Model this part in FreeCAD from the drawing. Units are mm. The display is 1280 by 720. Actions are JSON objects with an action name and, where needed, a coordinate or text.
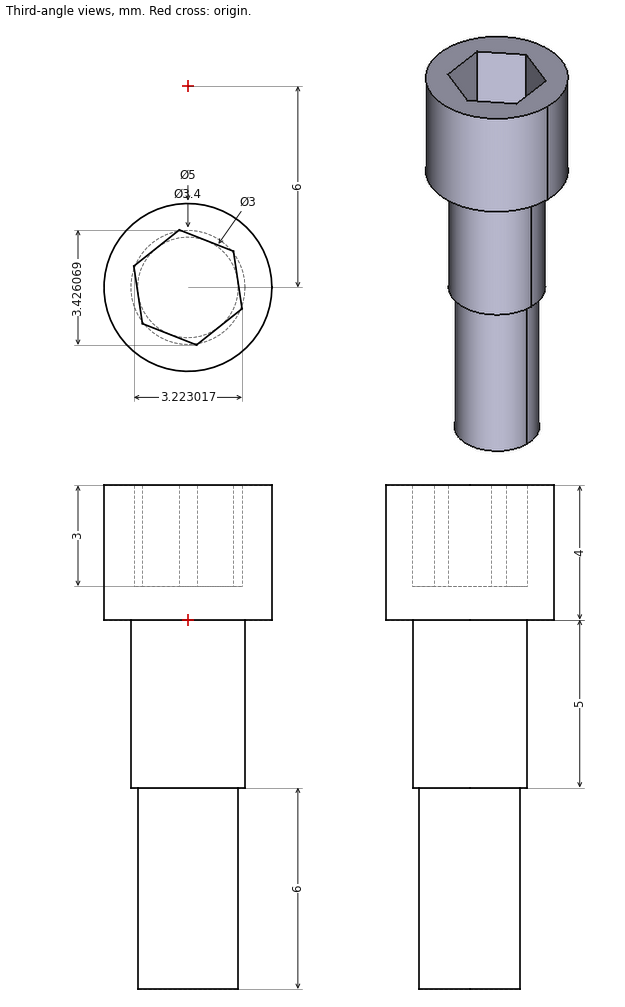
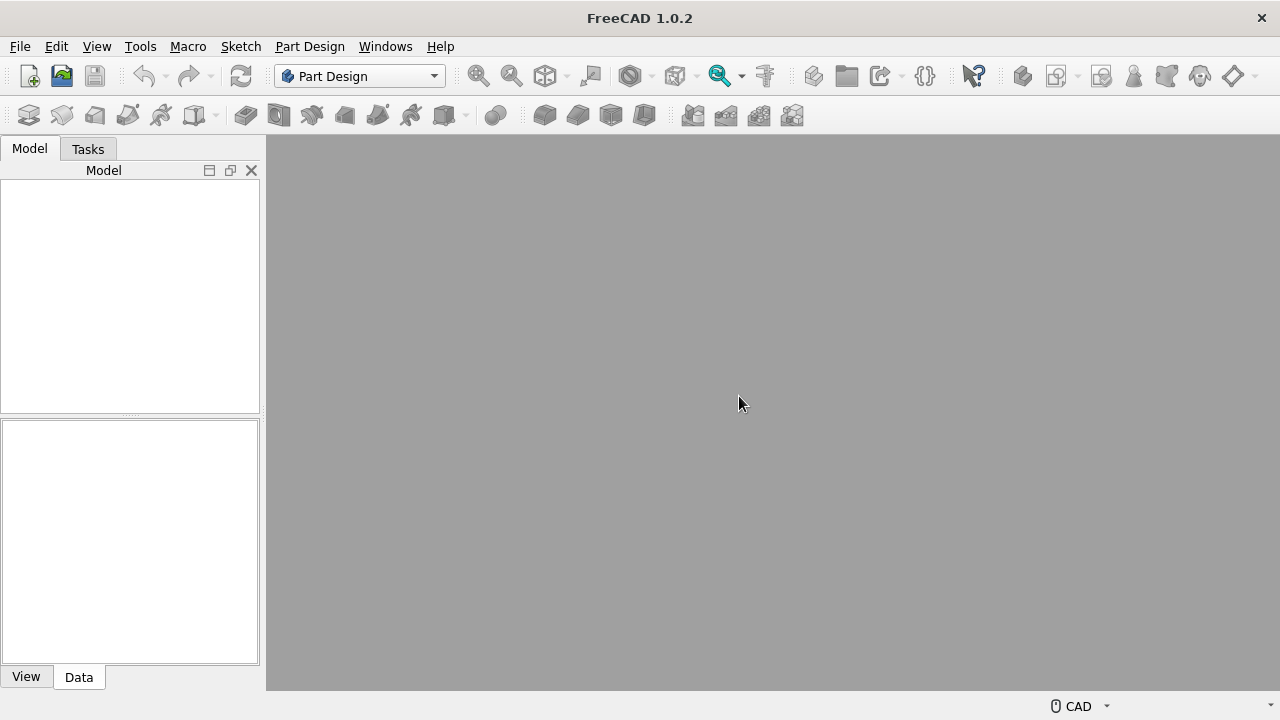
{"action": "left_click", "coordinate": [29, 76]}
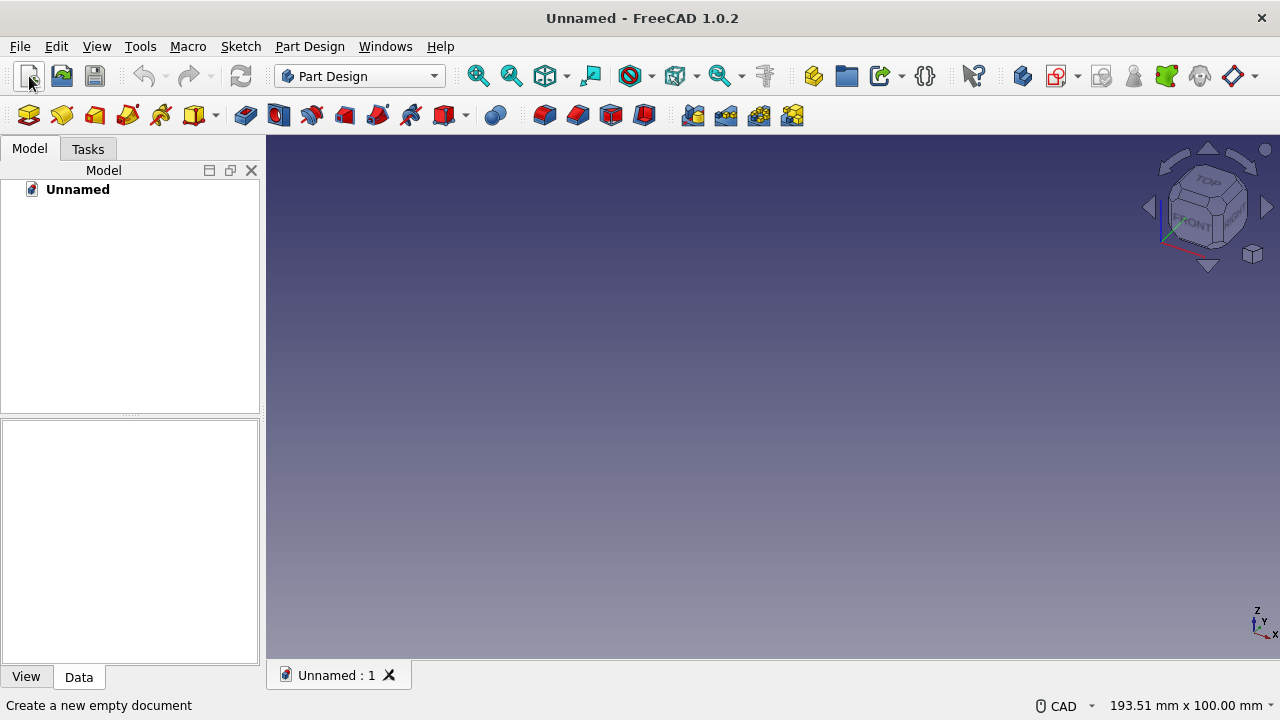
{"action": "left_click", "coordinate": [1056, 76]}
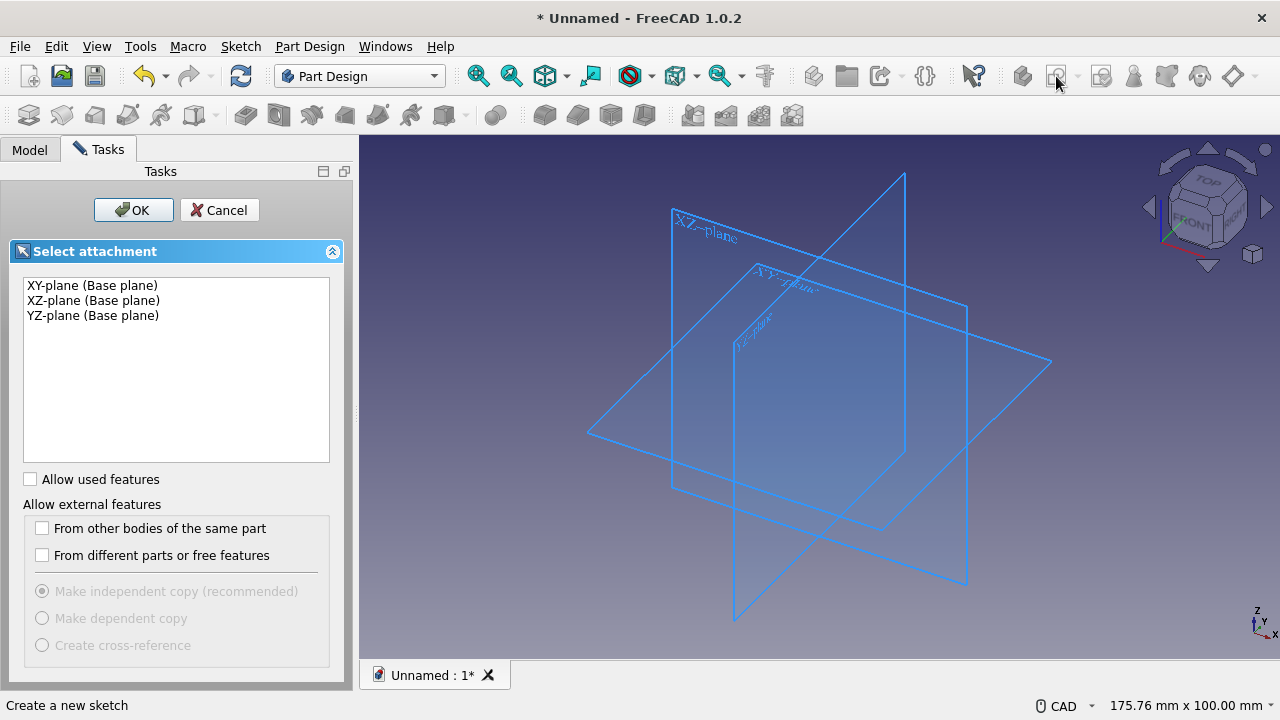
{"action": "left_click", "coordinate": [84, 286]}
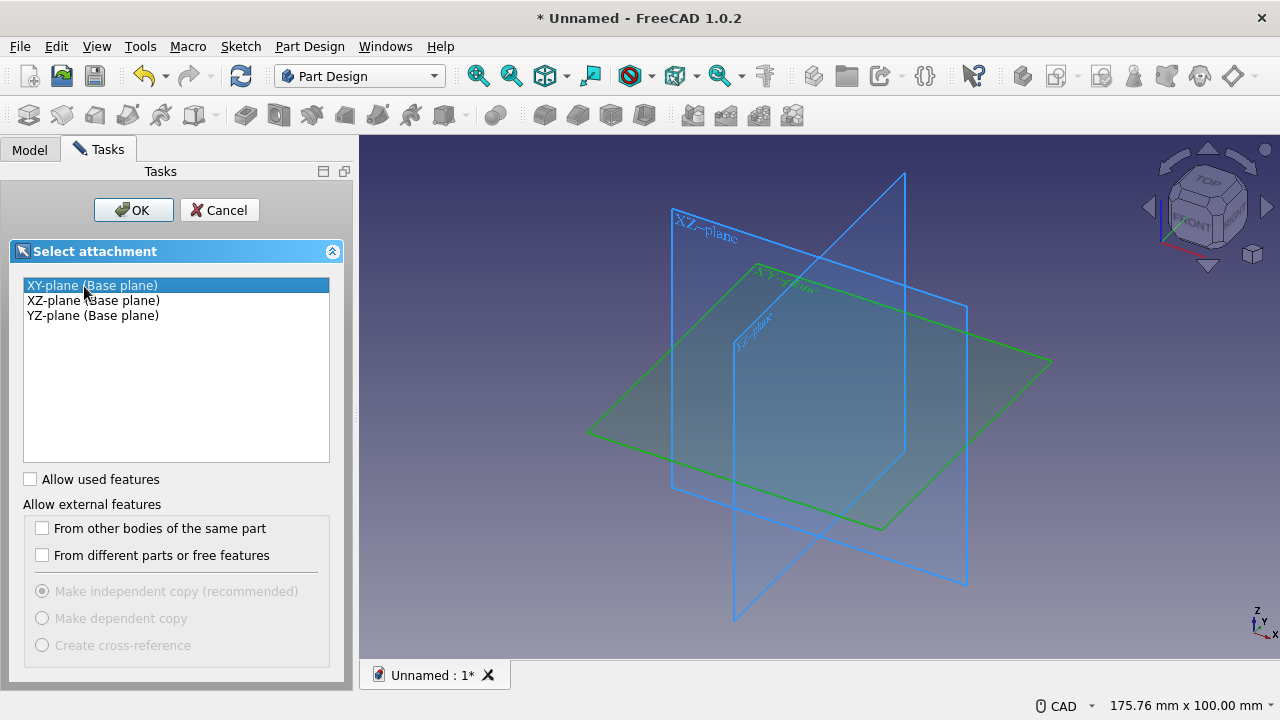
{"action": "left_click", "coordinate": [134, 210]}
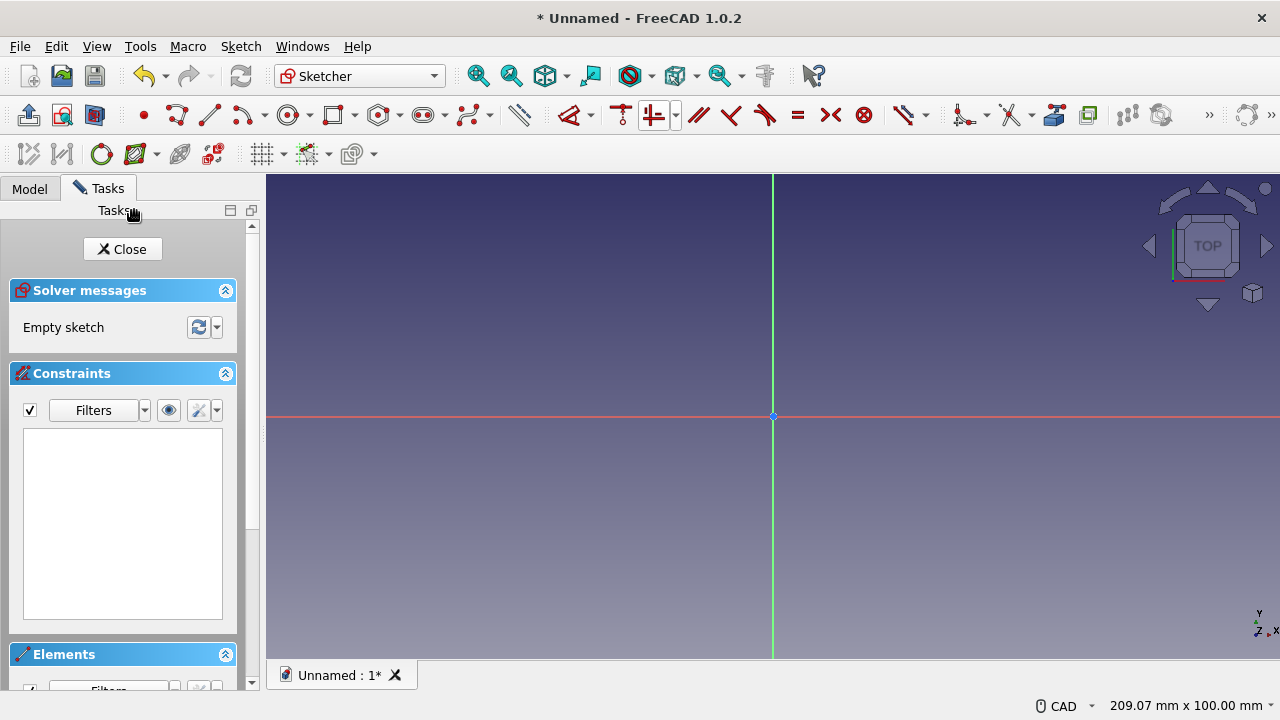
{"action": "scroll", "coordinate": [784, 438], "scroll_direction": "up", "scroll_amount": 10}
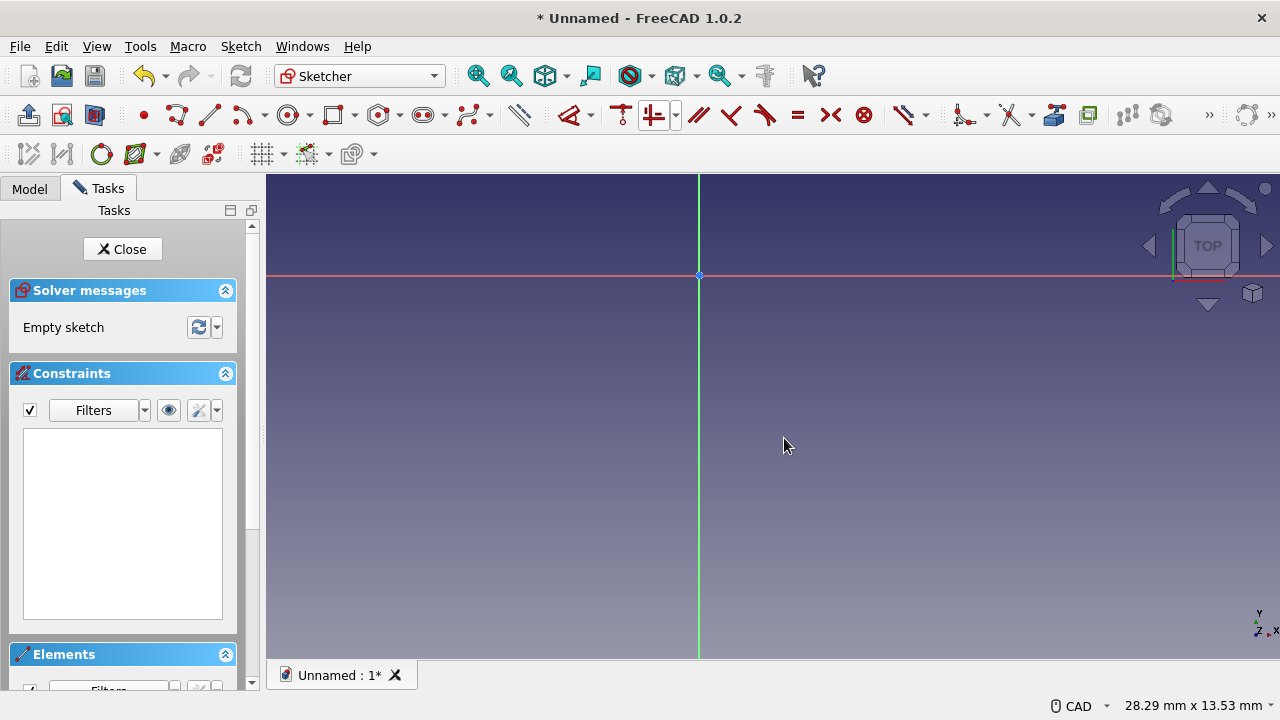
{"action": "key", "text": "g c"}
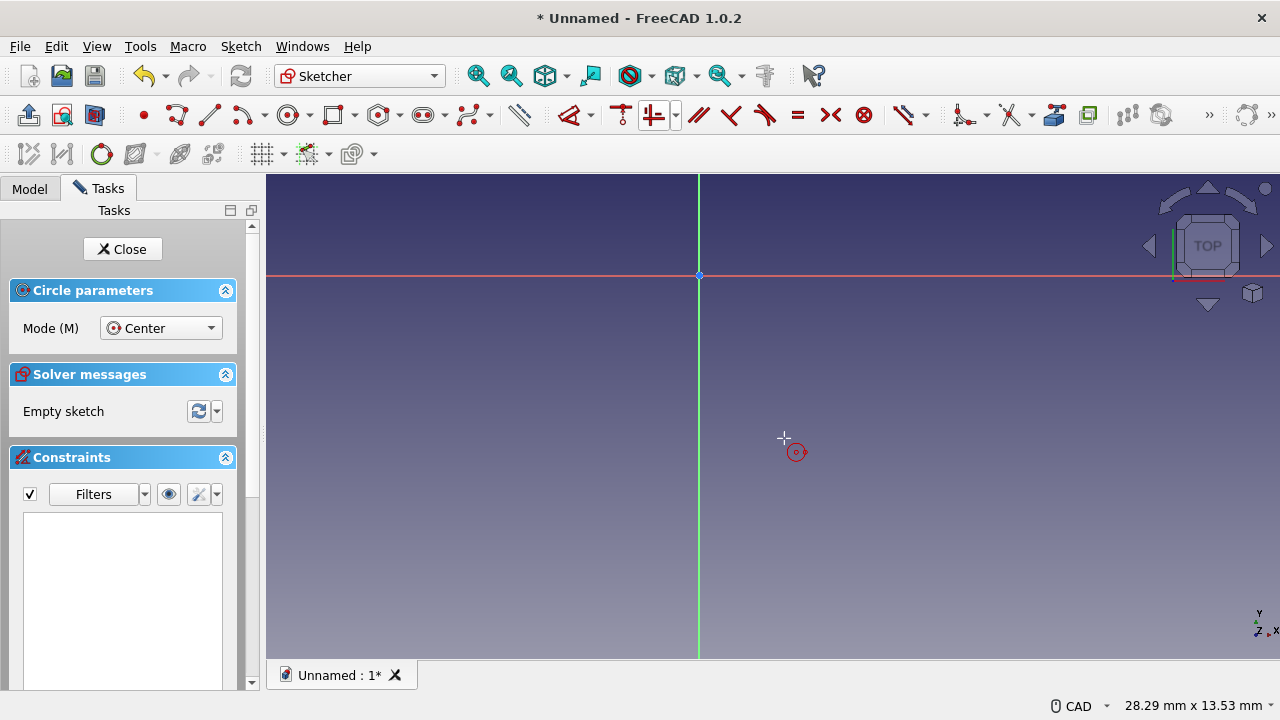
{"action": "left_click", "coordinate": [699, 491]}
{"action": "left_click", "coordinate": [743, 448]}
{"action": "key", "text": "Escape"}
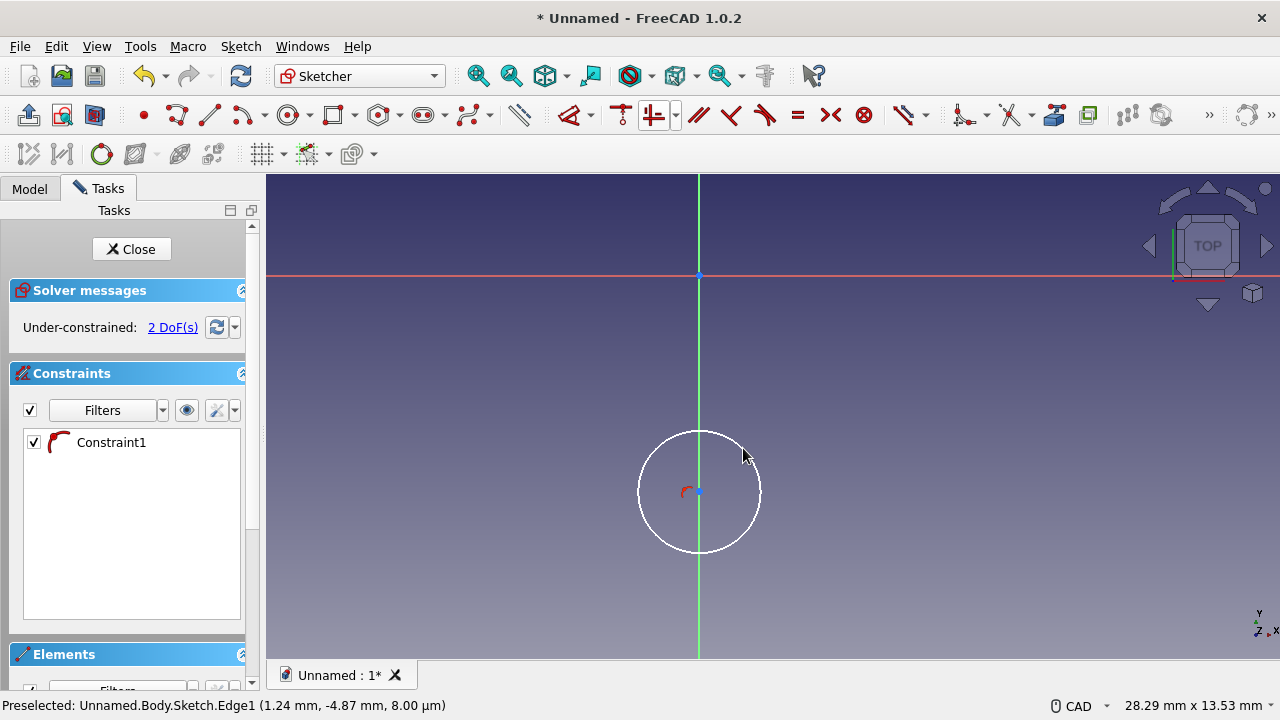
{"action": "key", "text": "d"}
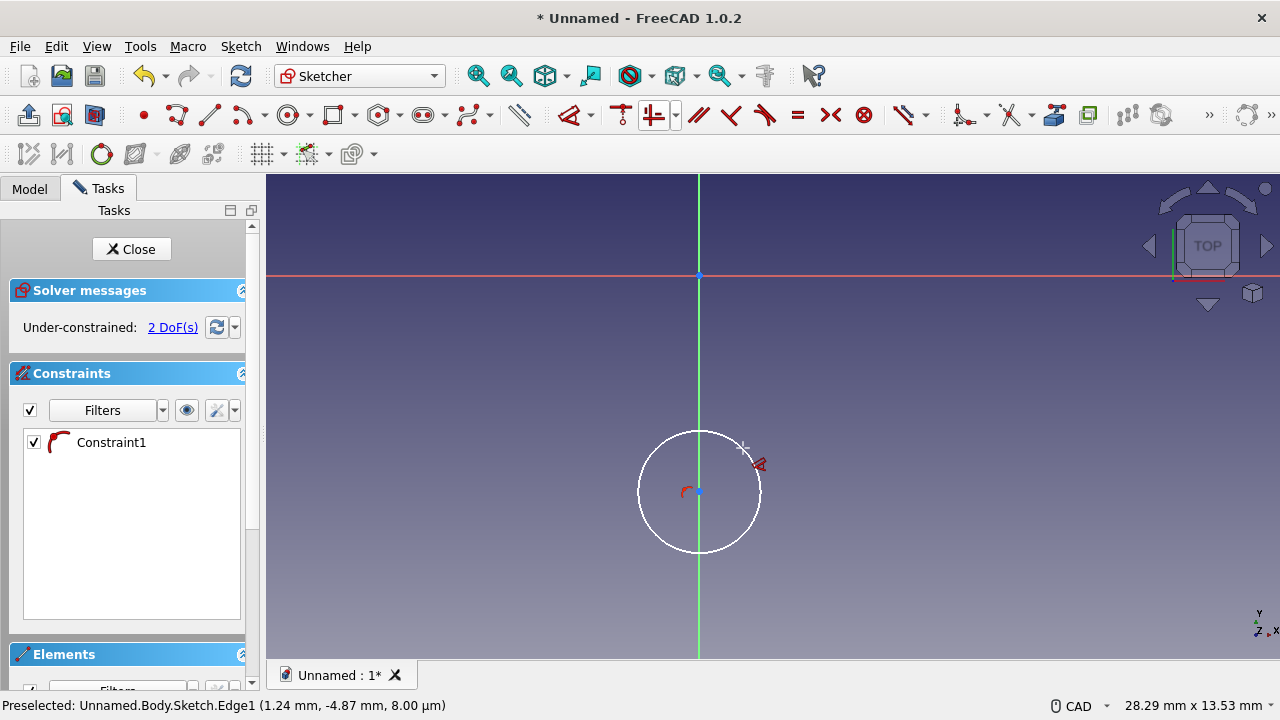
{"action": "left_click", "coordinate": [743, 449]}
{"action": "left_click", "coordinate": [766, 427]}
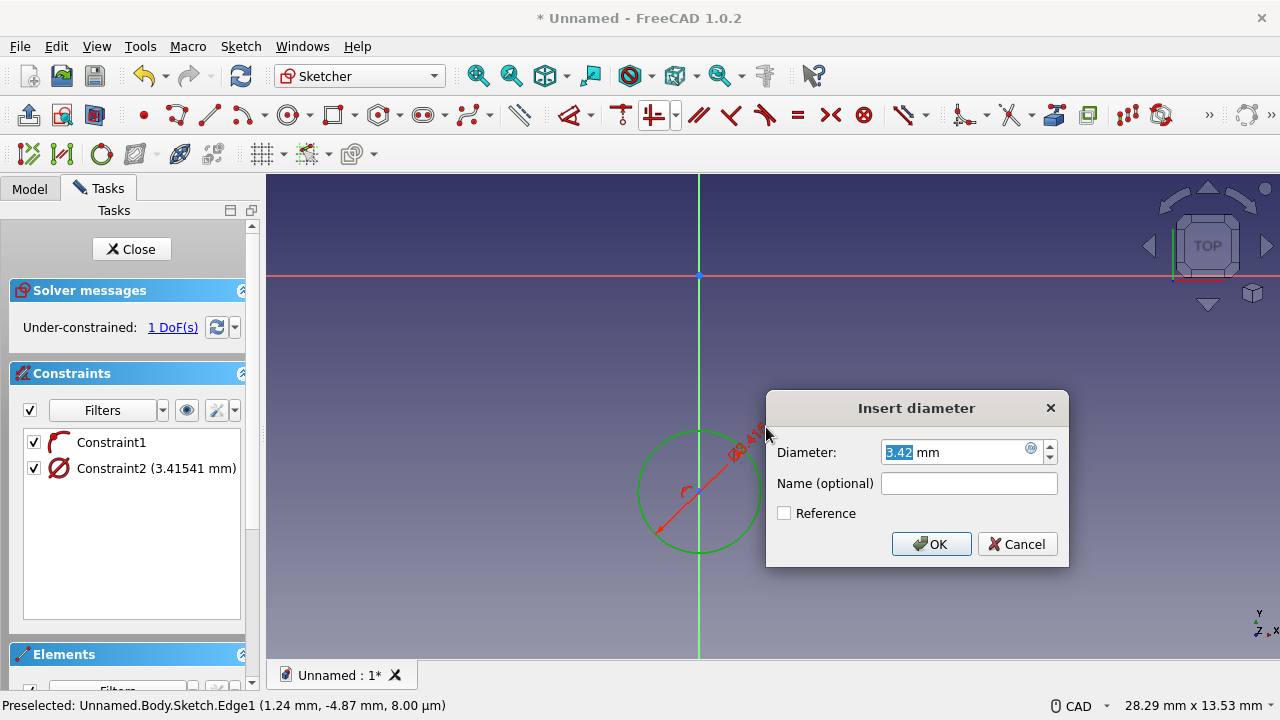
{"action": "type", "text": "3.4"}
{"action": "key", "text": "Return"}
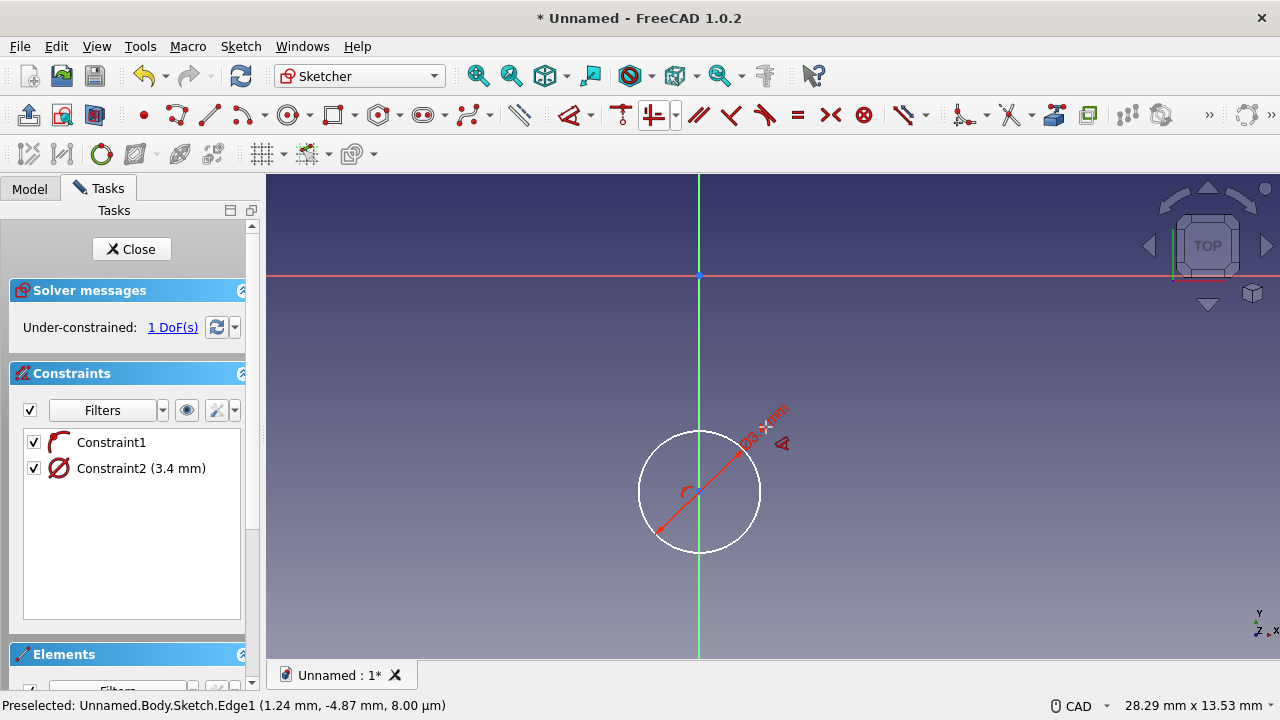
{"action": "left_click", "coordinate": [699, 492]}
{"action": "left_click", "coordinate": [733, 384]}